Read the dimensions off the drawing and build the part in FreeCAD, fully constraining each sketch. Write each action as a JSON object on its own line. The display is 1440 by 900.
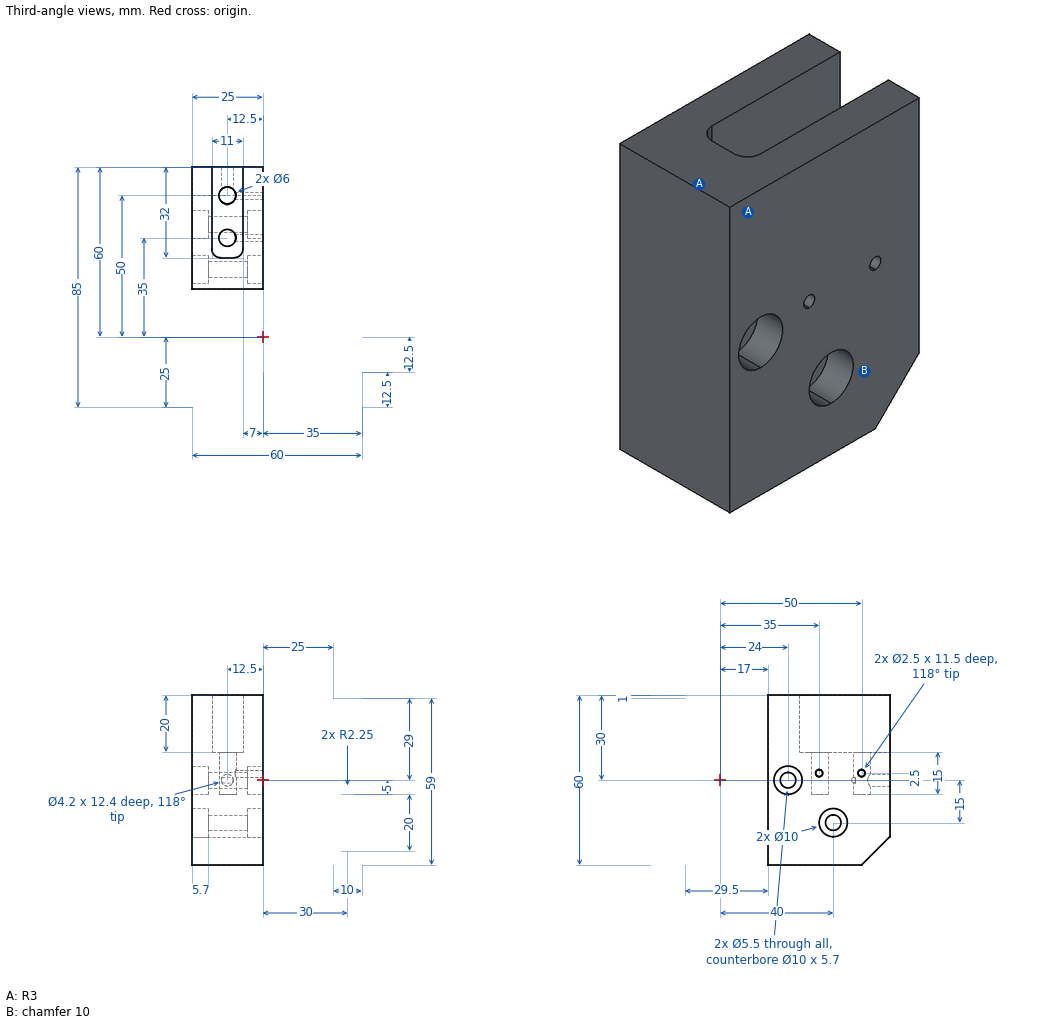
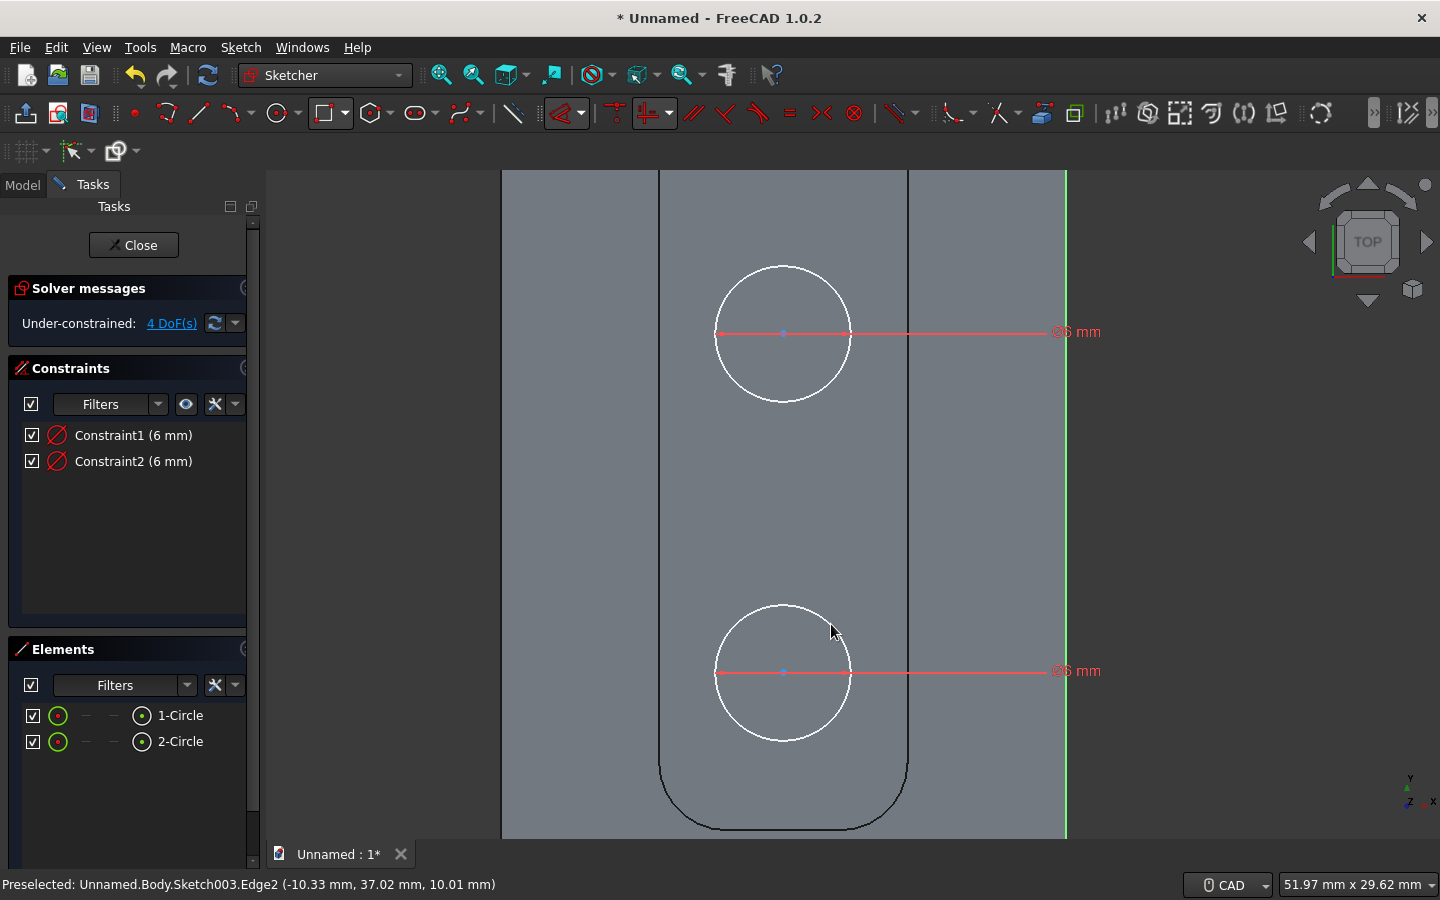
{"action": "left_click", "coordinate": [783, 334]}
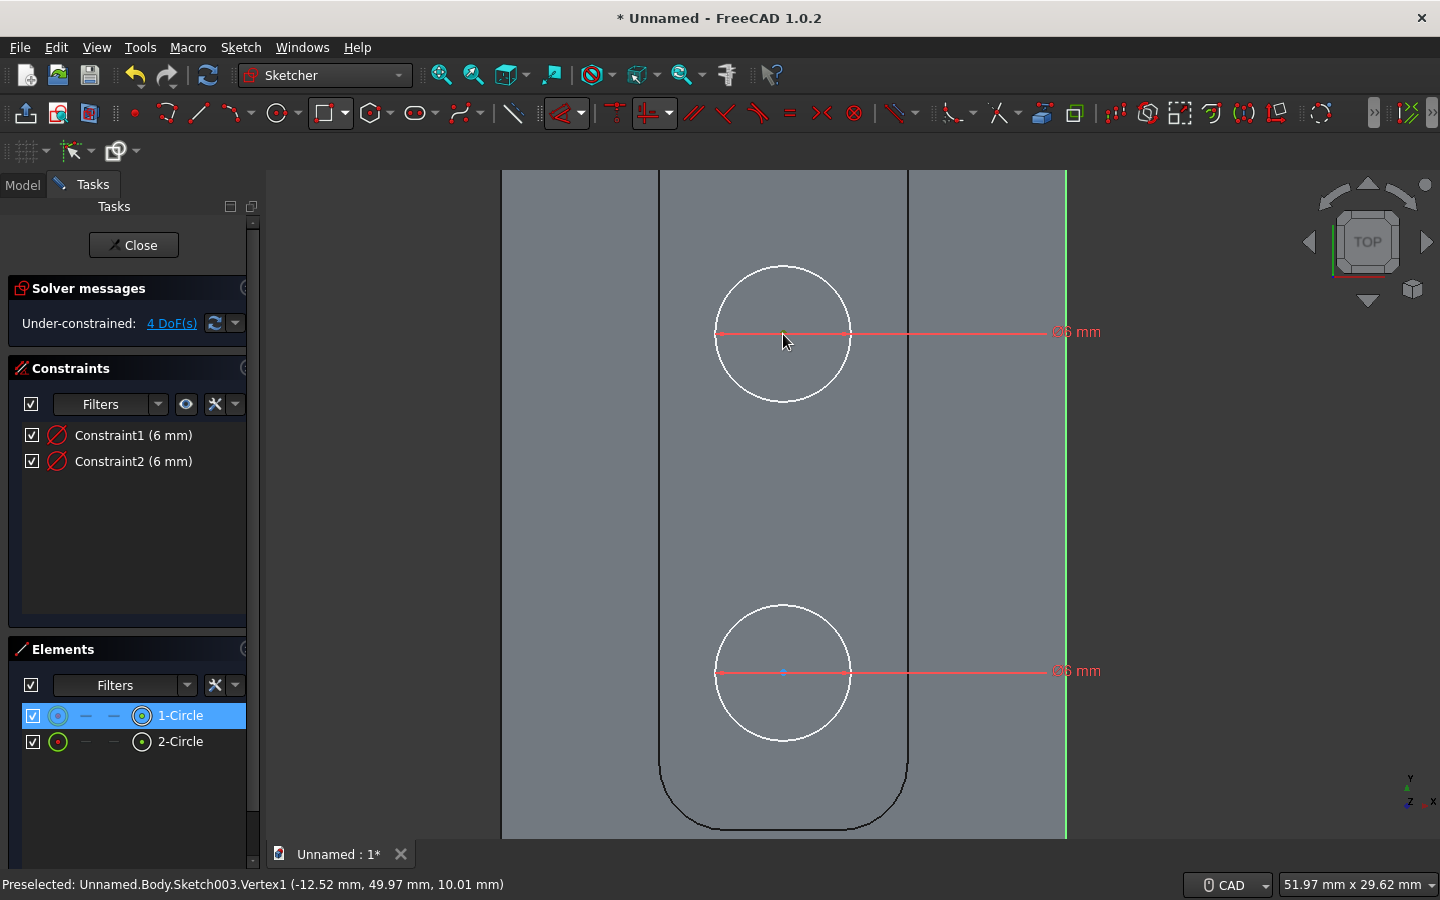
{"action": "left_click", "coordinate": [783, 673]}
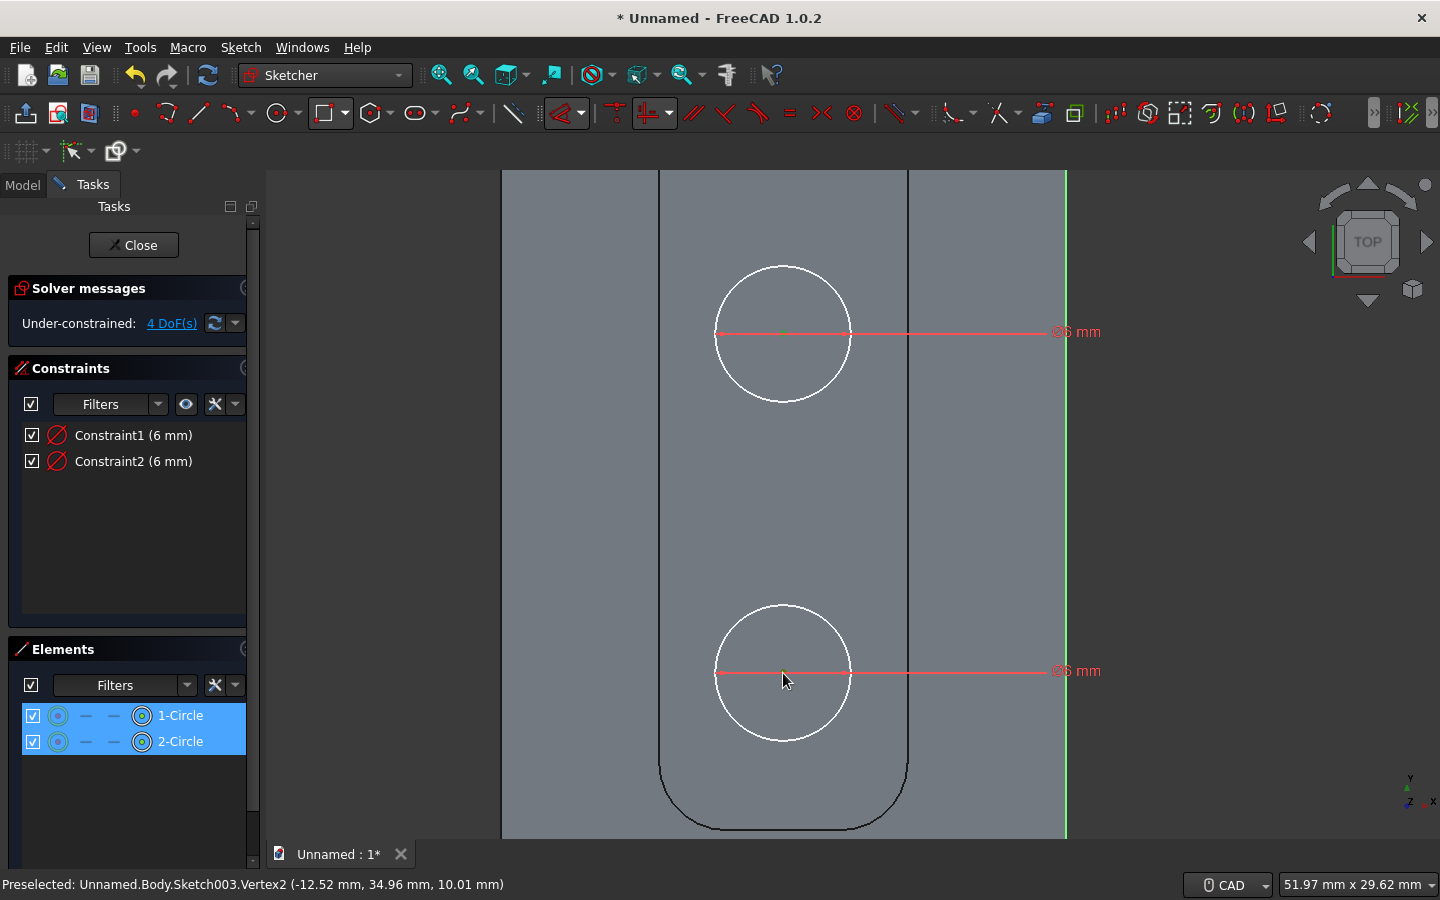
{"action": "left_click", "coordinate": [672, 114]}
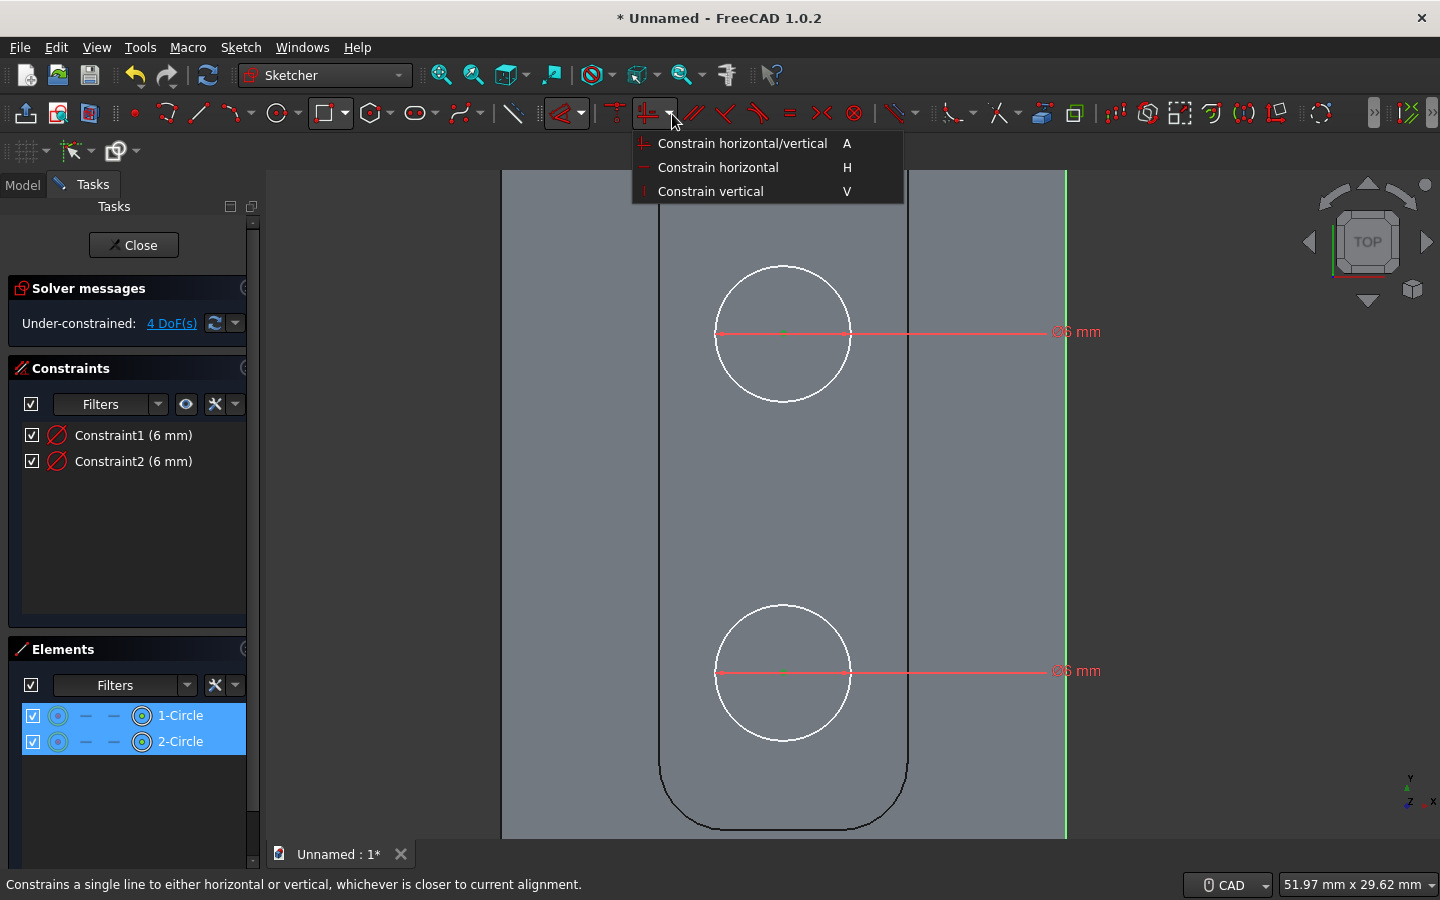
{"action": "left_click", "coordinate": [768, 191]}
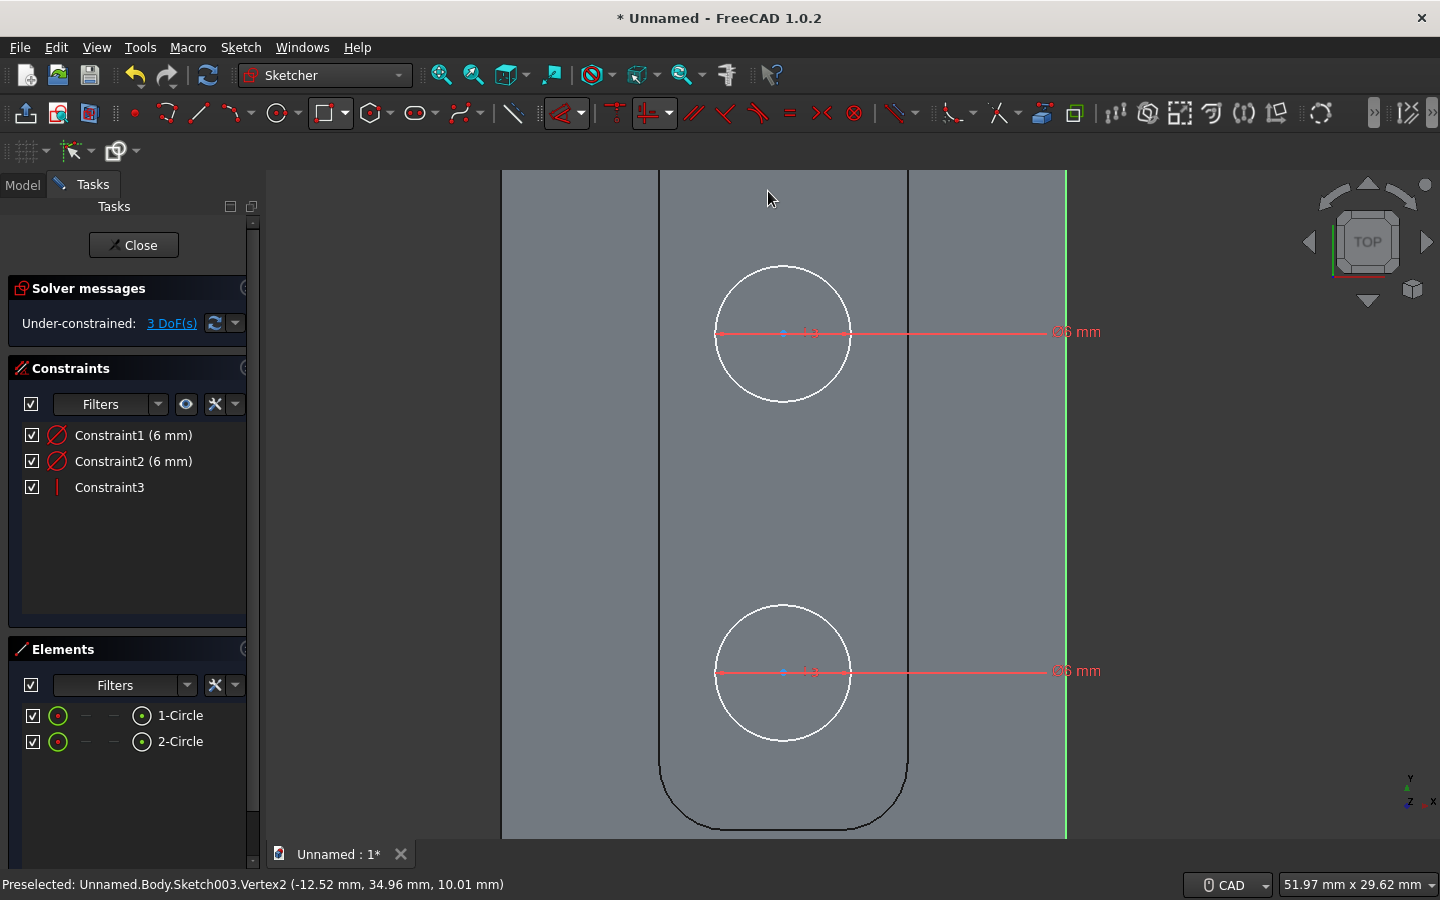
{"action": "left_click", "coordinate": [783, 334]}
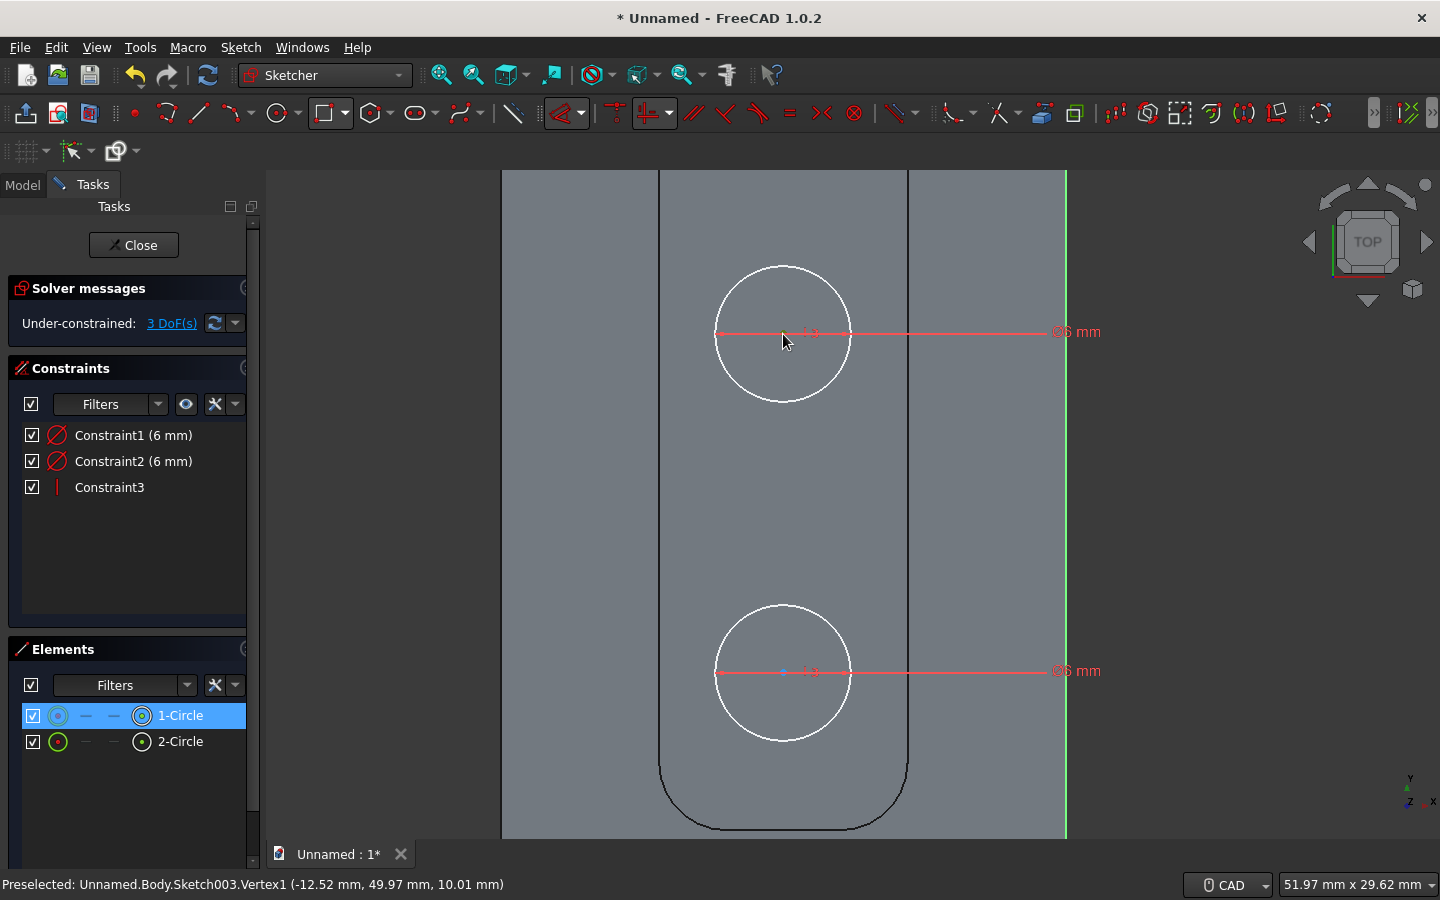
{"action": "left_click", "coordinate": [584, 114]}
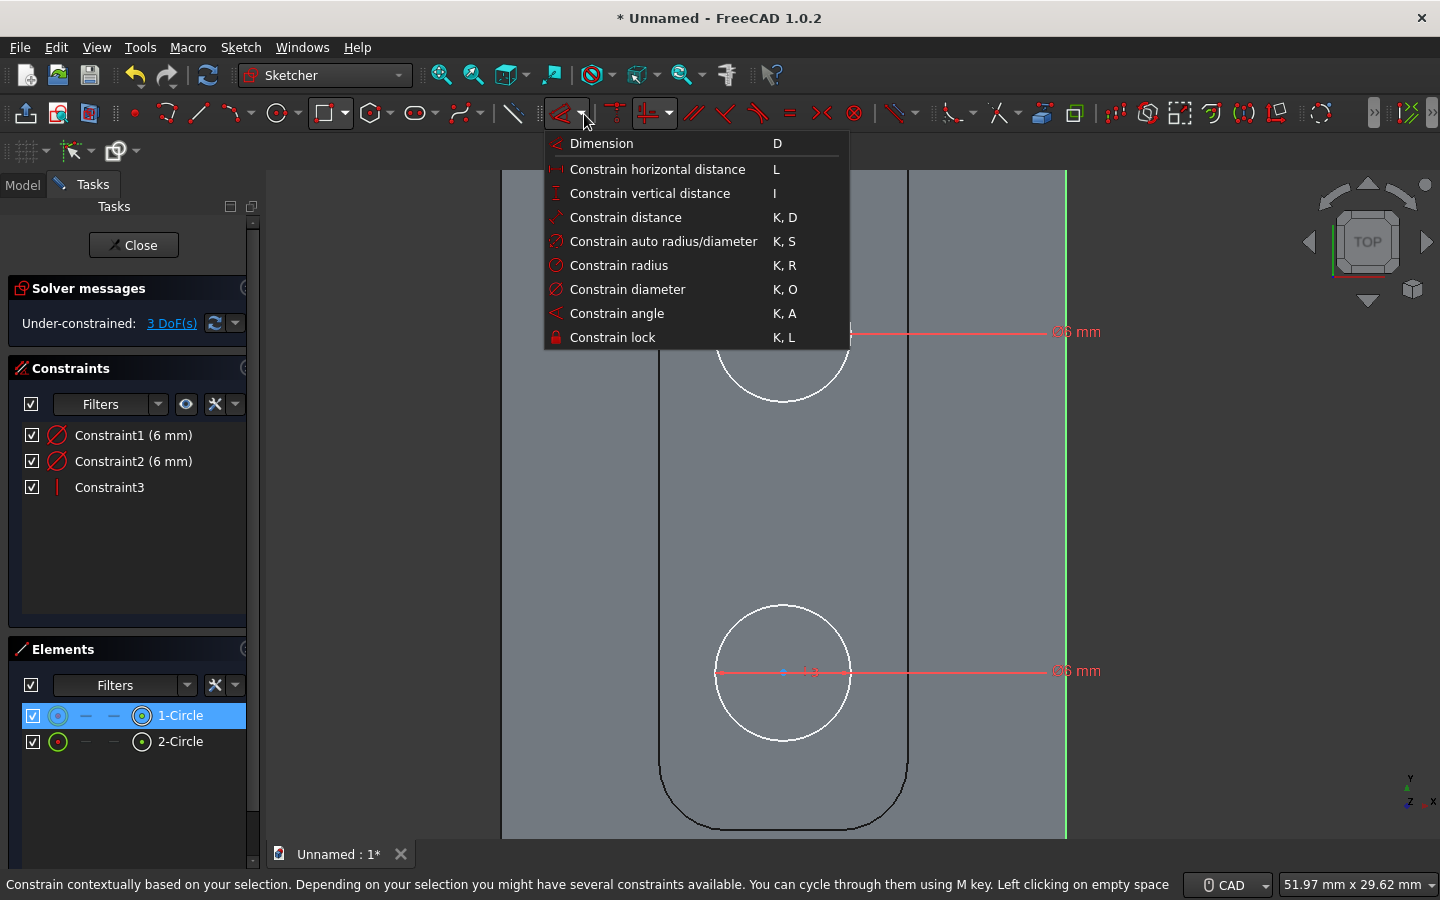
{"action": "left_click", "coordinate": [697, 193]}